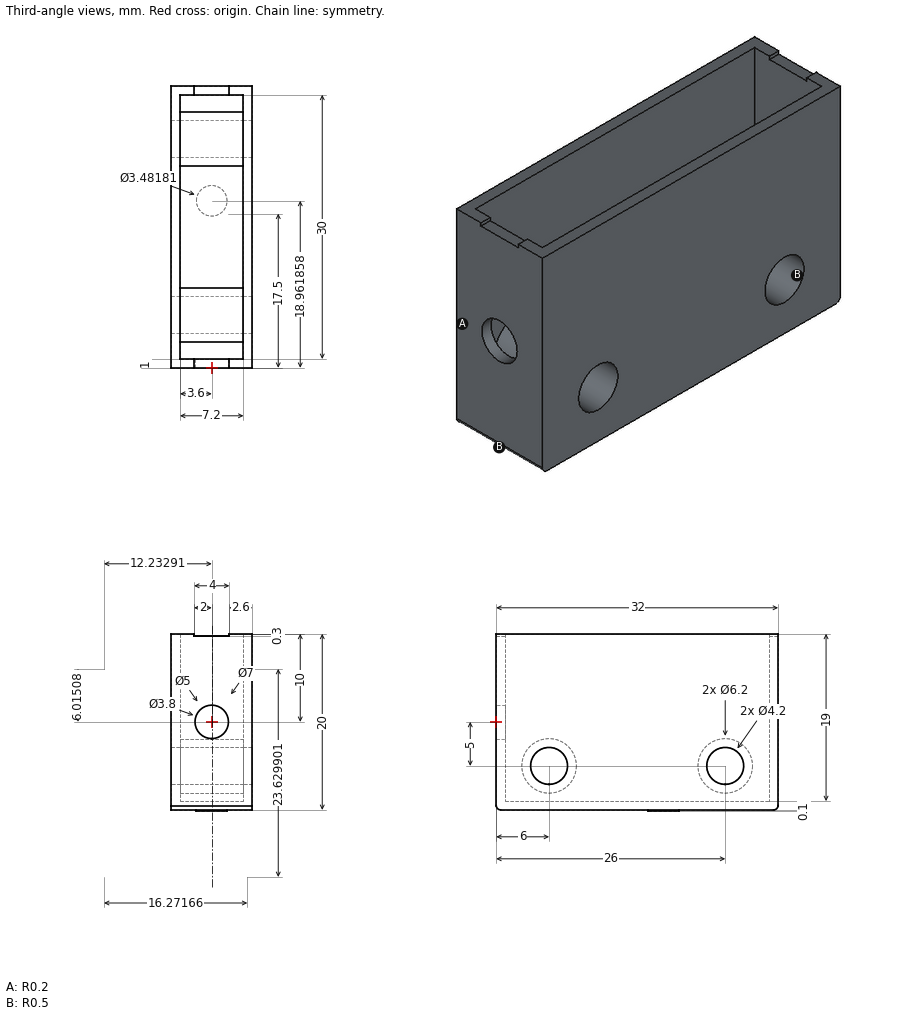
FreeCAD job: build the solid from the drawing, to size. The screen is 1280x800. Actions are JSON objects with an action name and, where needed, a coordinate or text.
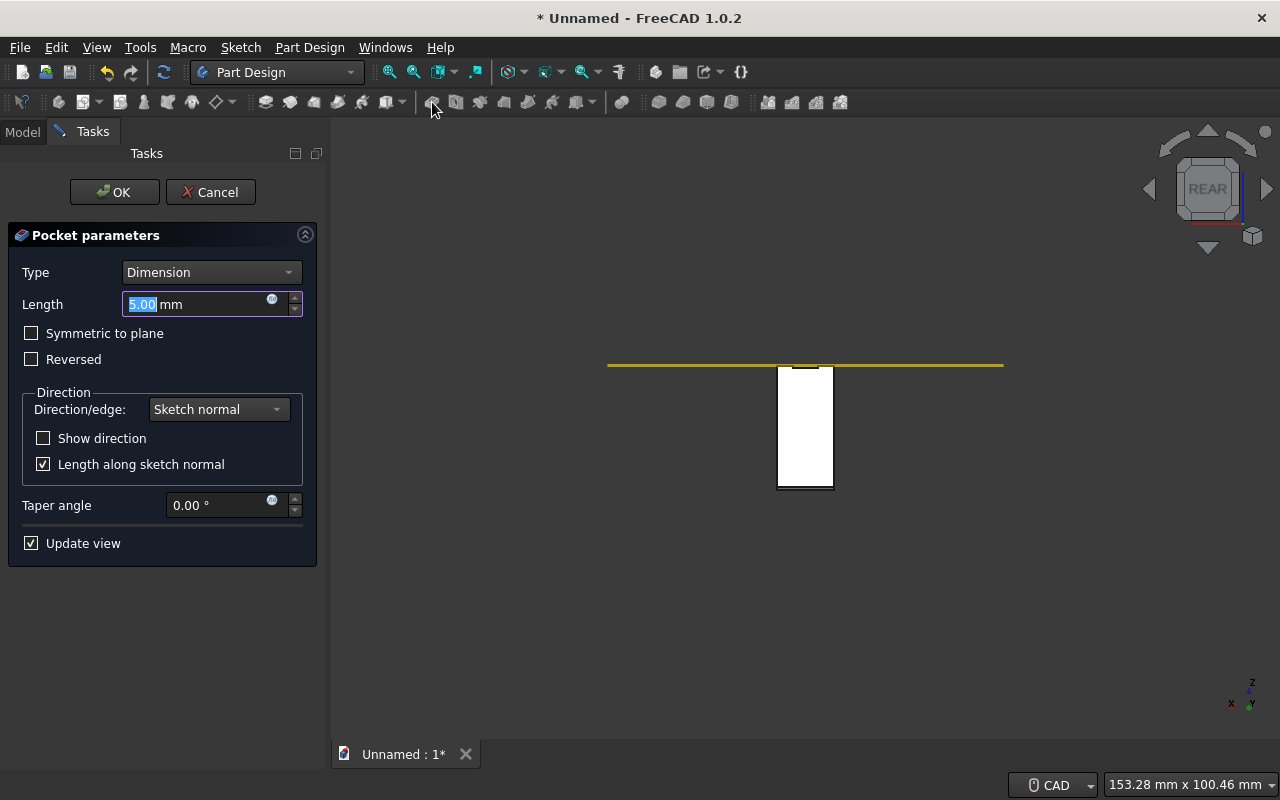
{"action": "type", "text": "19"}
{"action": "key", "text": "Tab"}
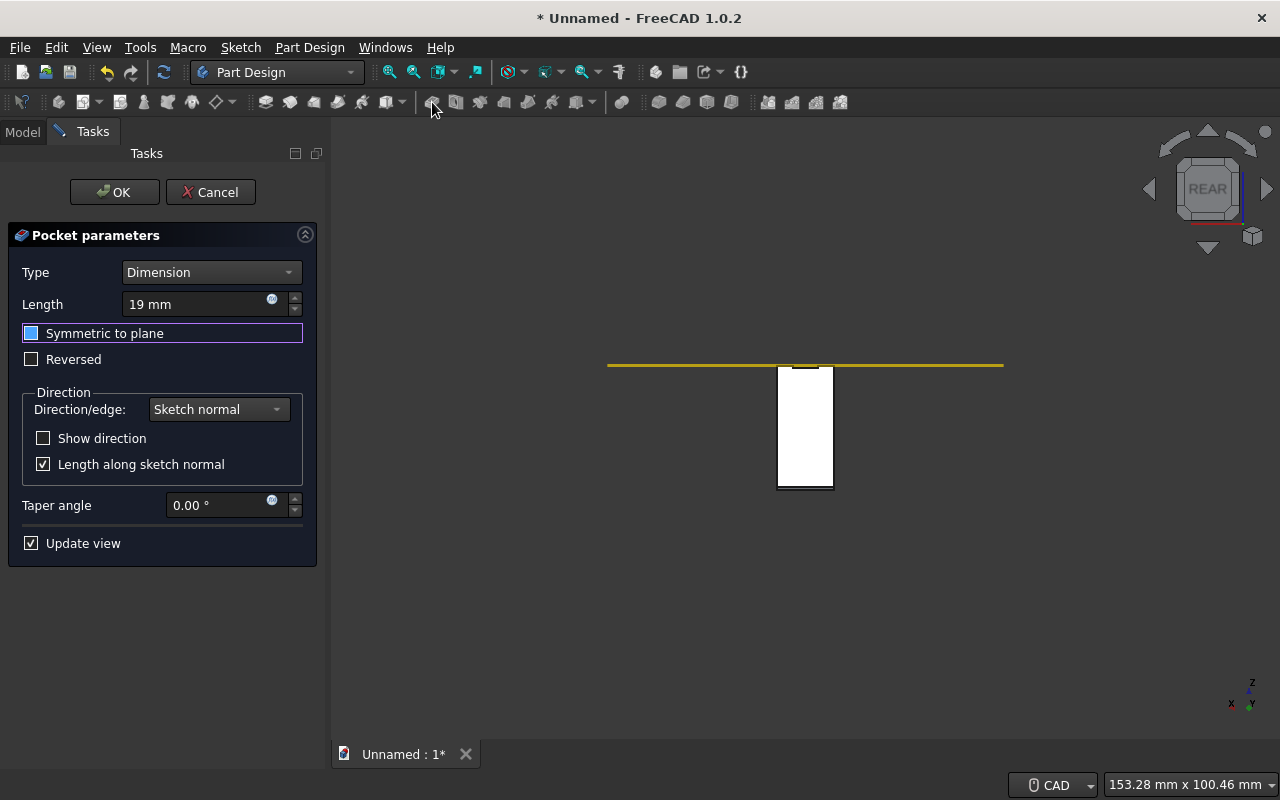
{"action": "left_click", "coordinate": [115, 192]}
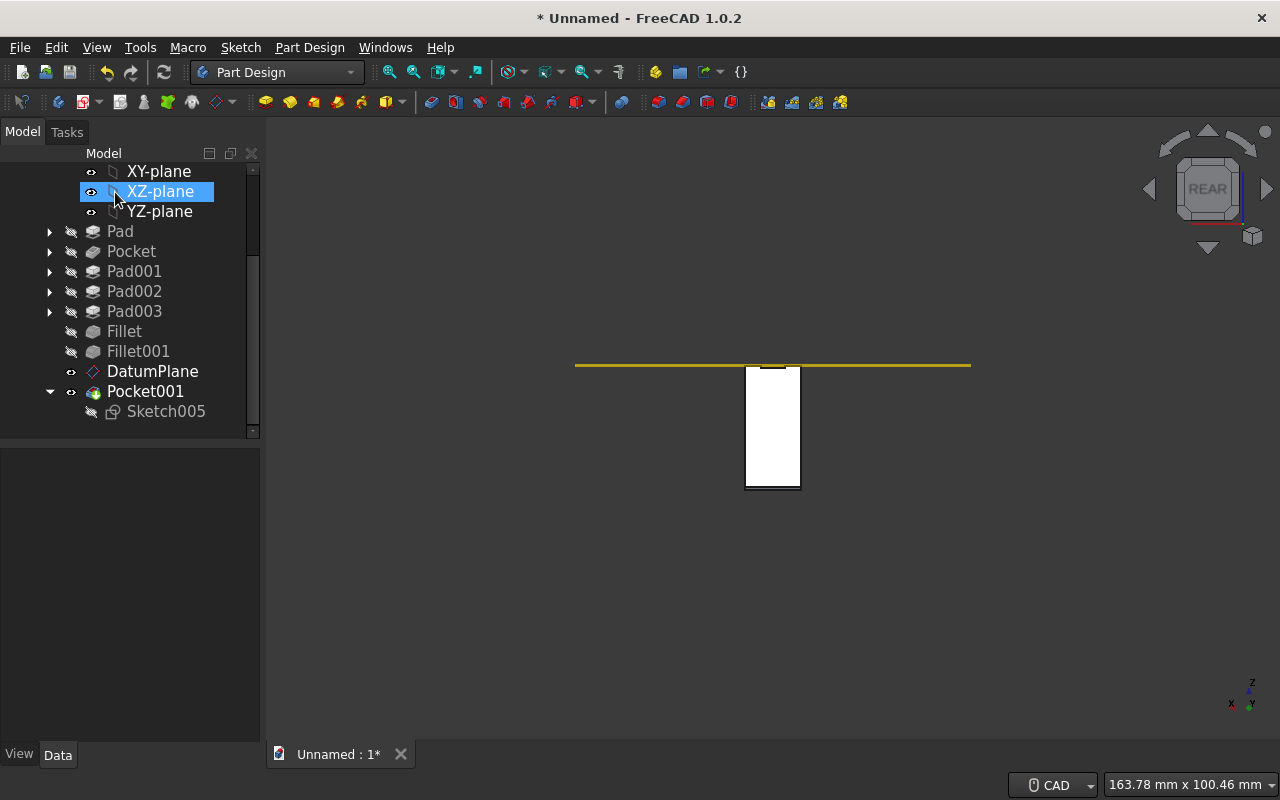
{"action": "left_click", "coordinate": [116, 372]}
{"action": "key", "text": "space"}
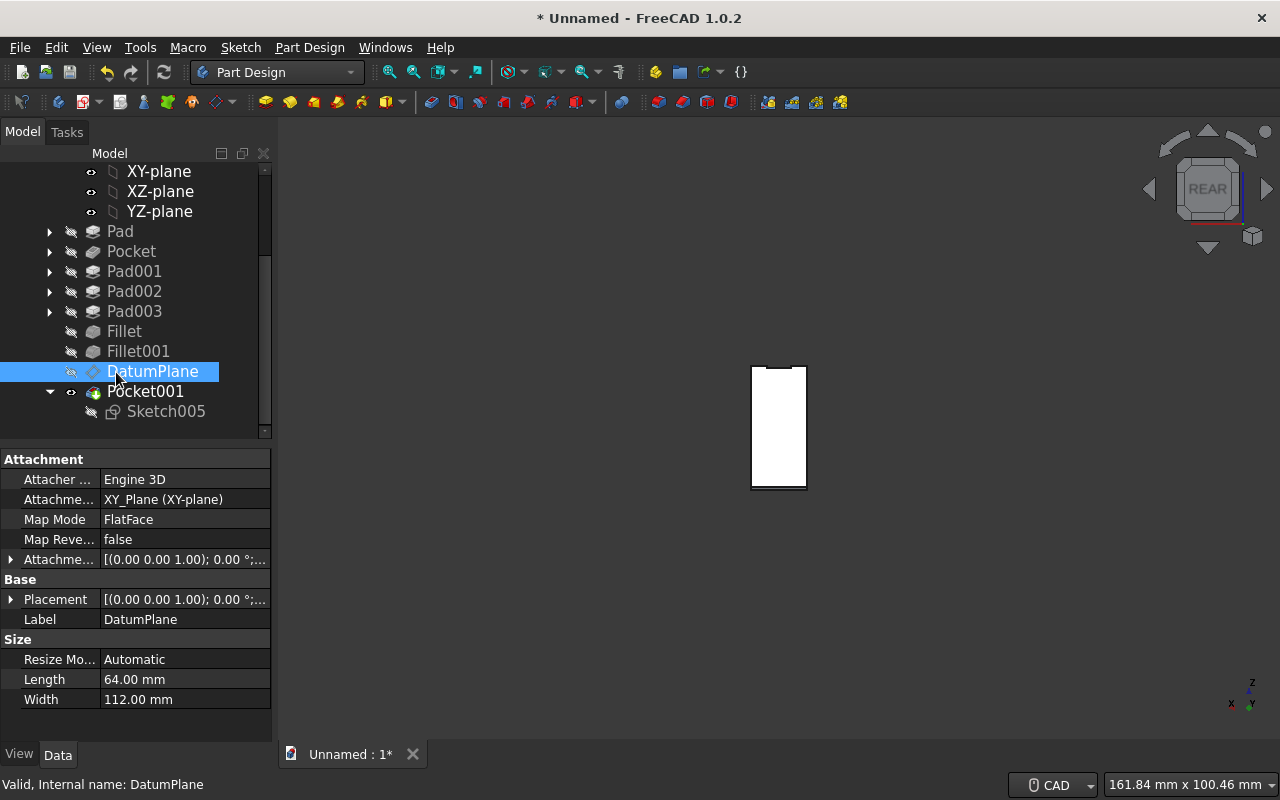
{"action": "left_click", "coordinate": [390, 72]}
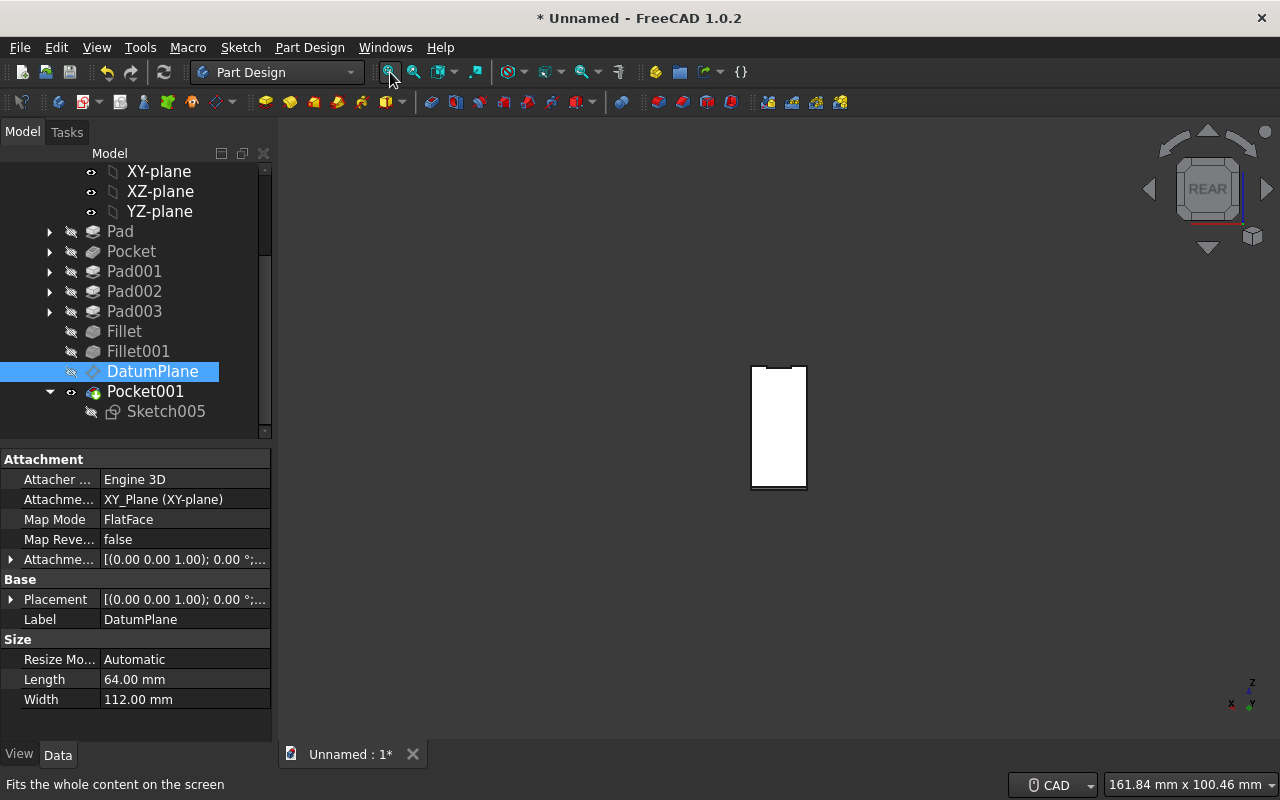
{"action": "key", "text": "0"}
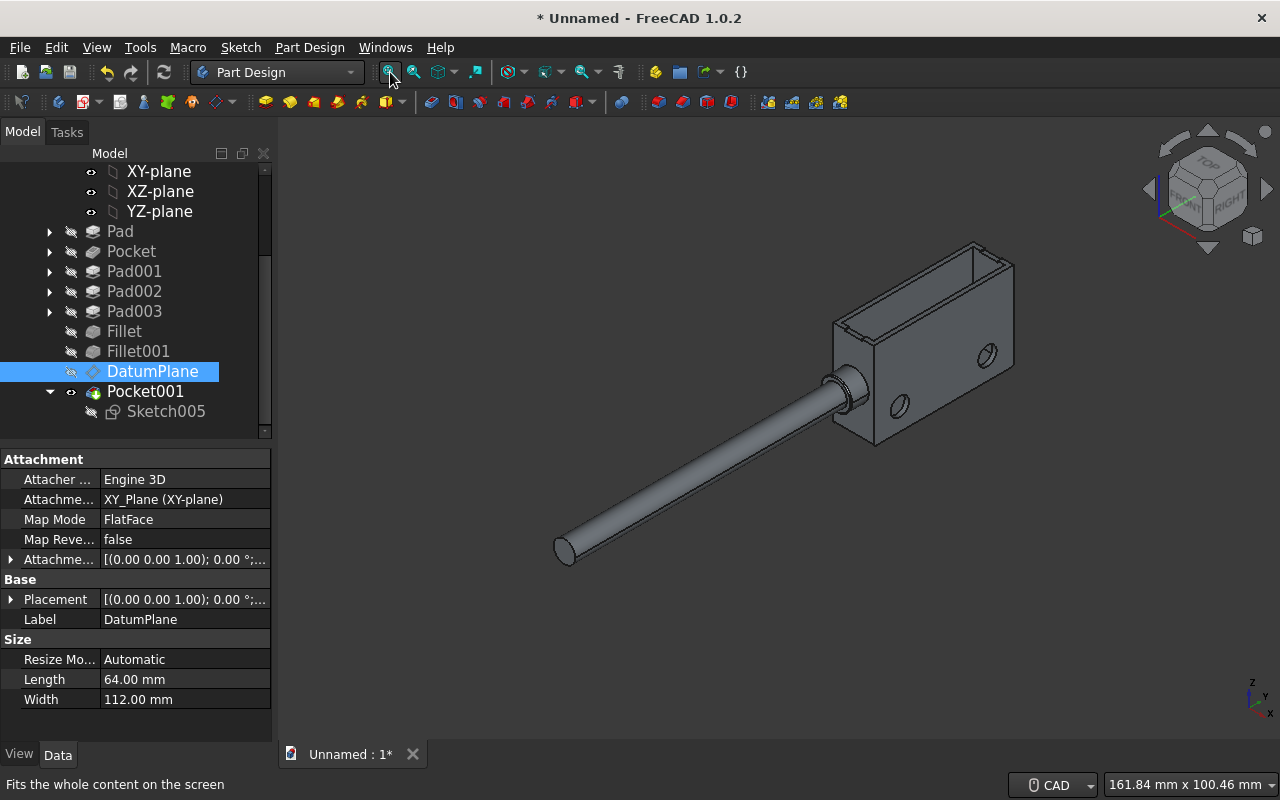
{"action": "left_click", "coordinate": [859, 358]}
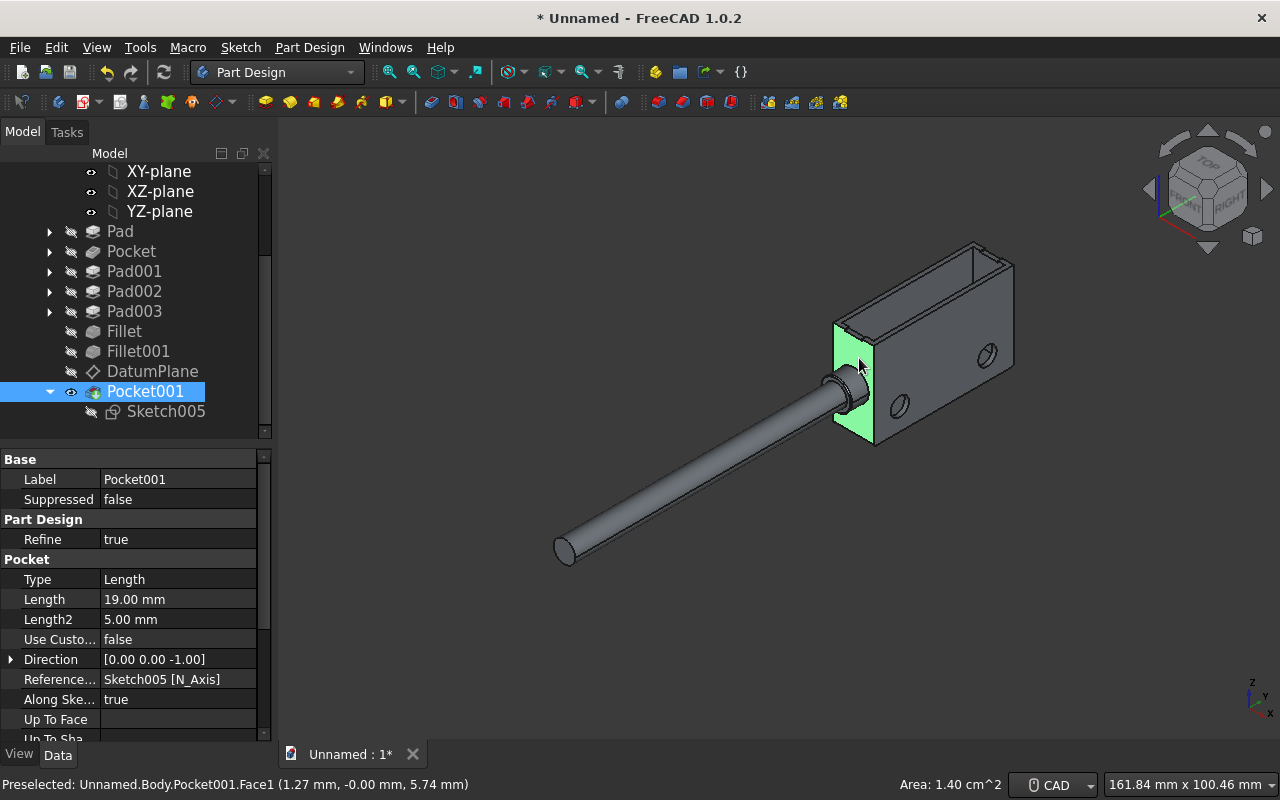
{"action": "left_click", "coordinate": [84, 102]}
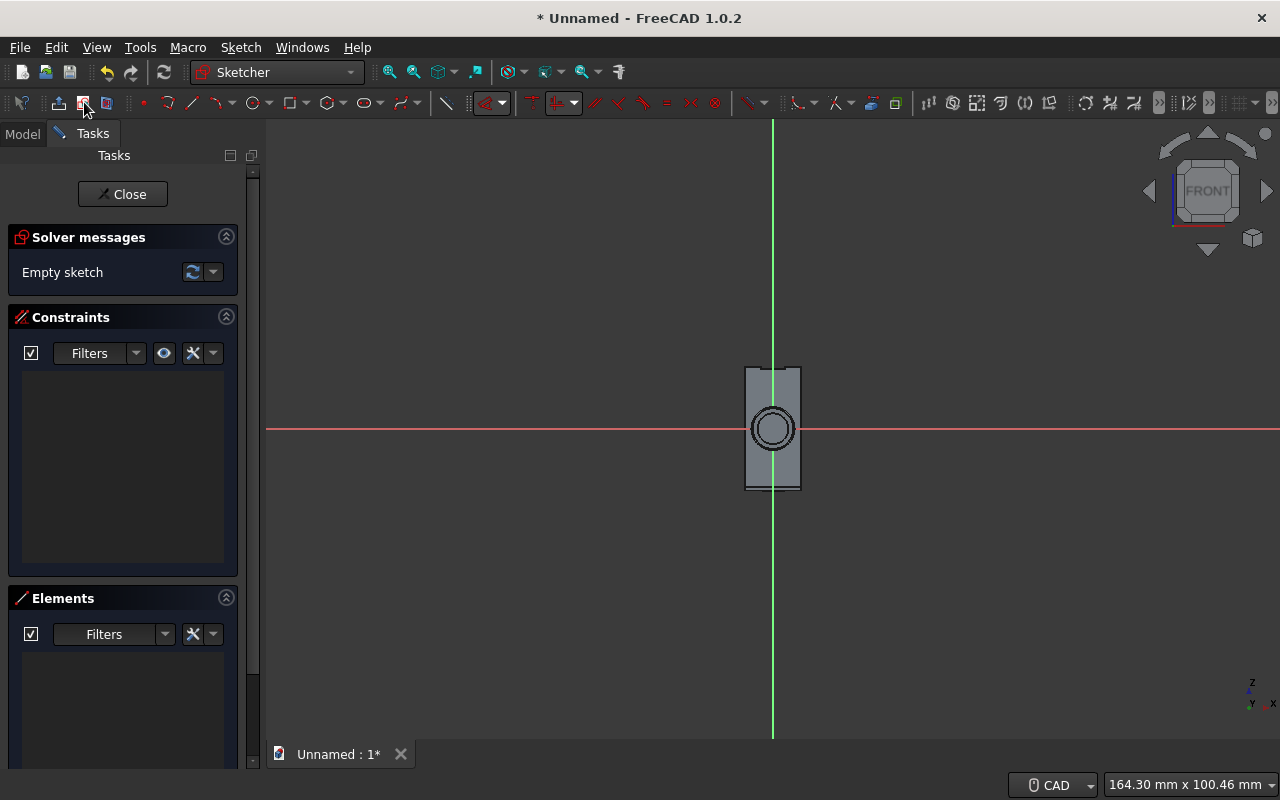
{"action": "left_click", "coordinate": [108, 104]}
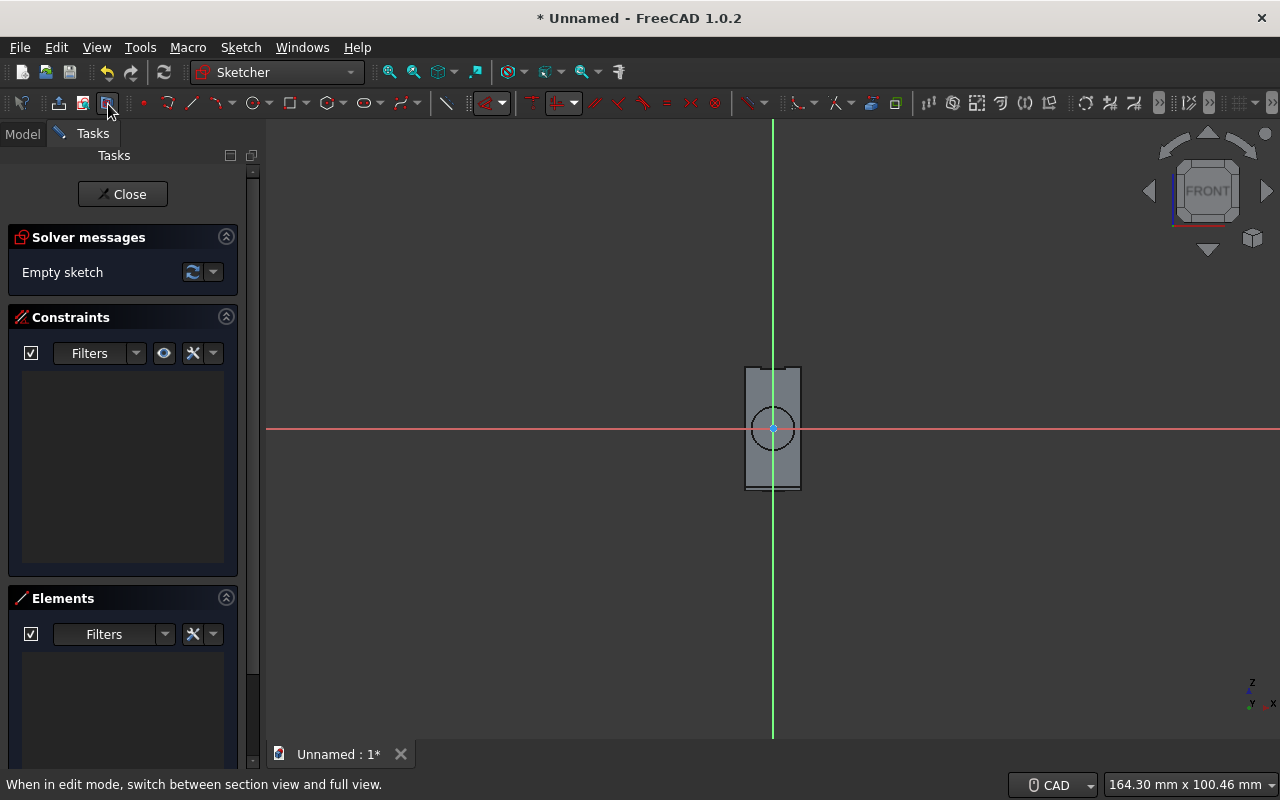
{"action": "scroll", "coordinate": [773, 485], "scroll_direction": "up", "scroll_amount": 5}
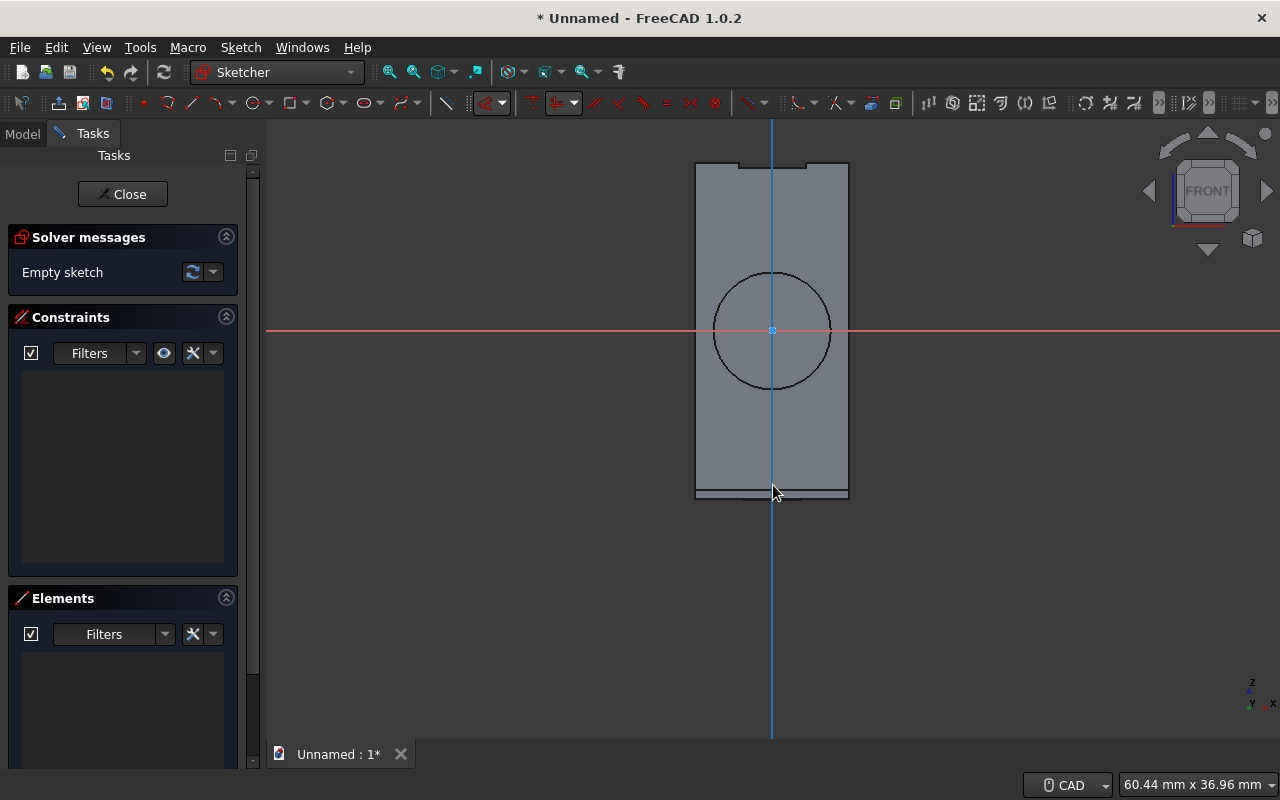
{"action": "left_click", "coordinate": [290, 104]}